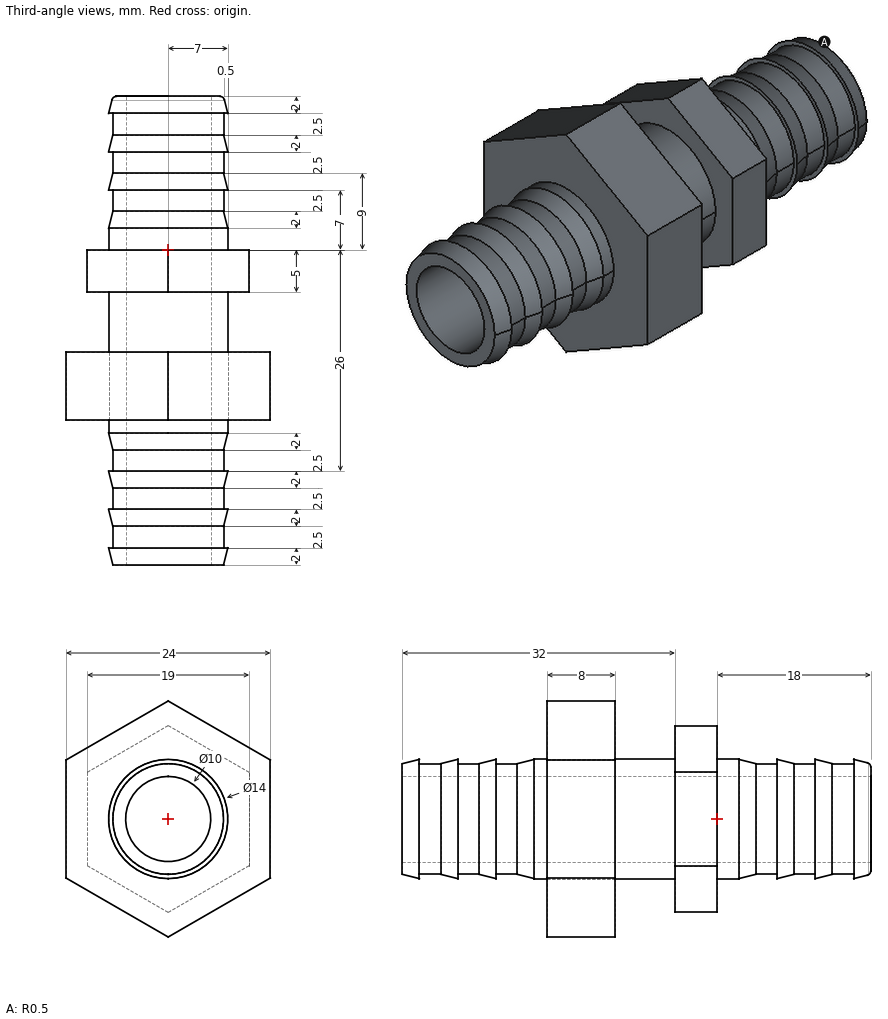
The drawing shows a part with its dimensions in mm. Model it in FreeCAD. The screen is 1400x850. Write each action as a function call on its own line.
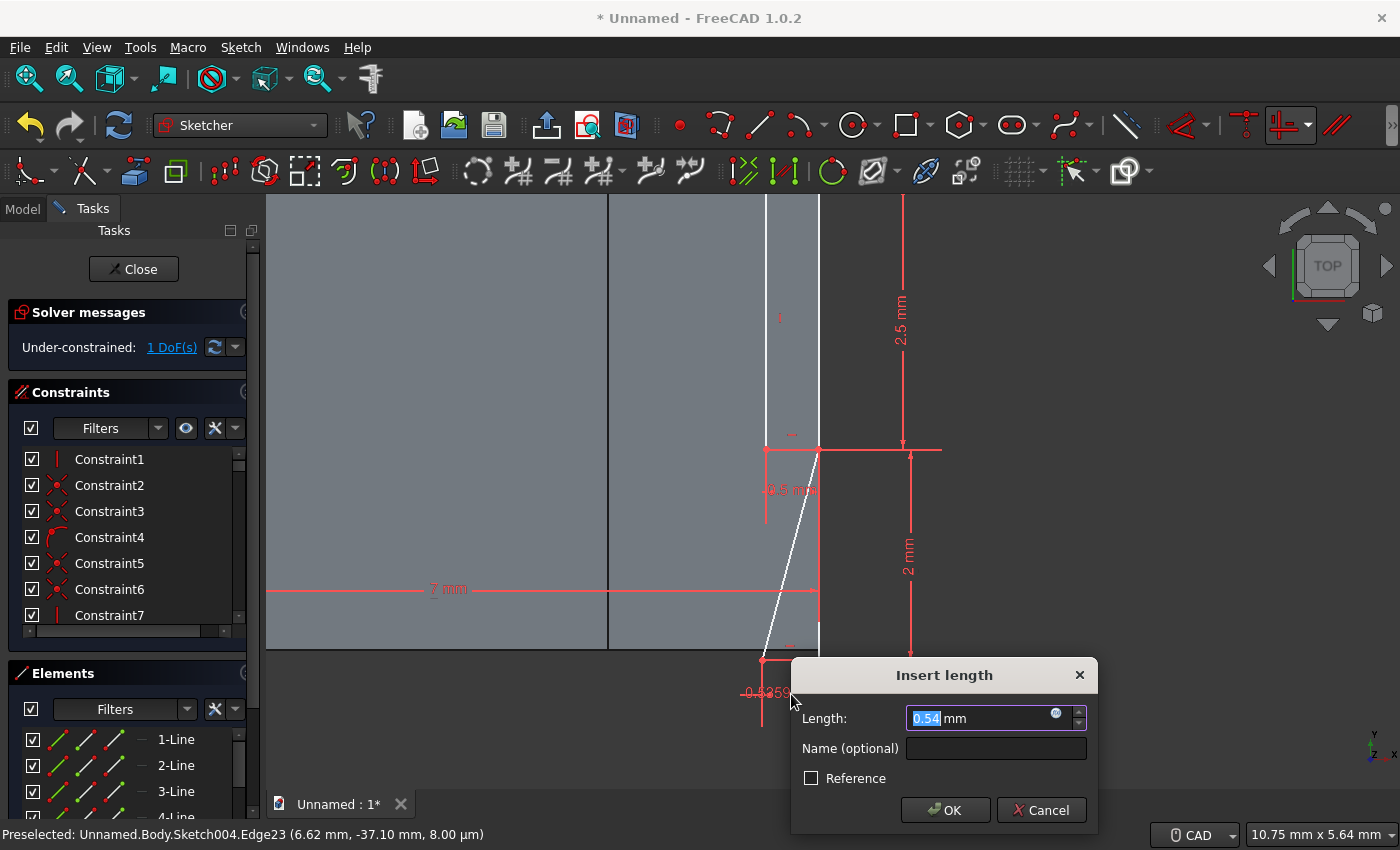
text(0.5)
key(Return)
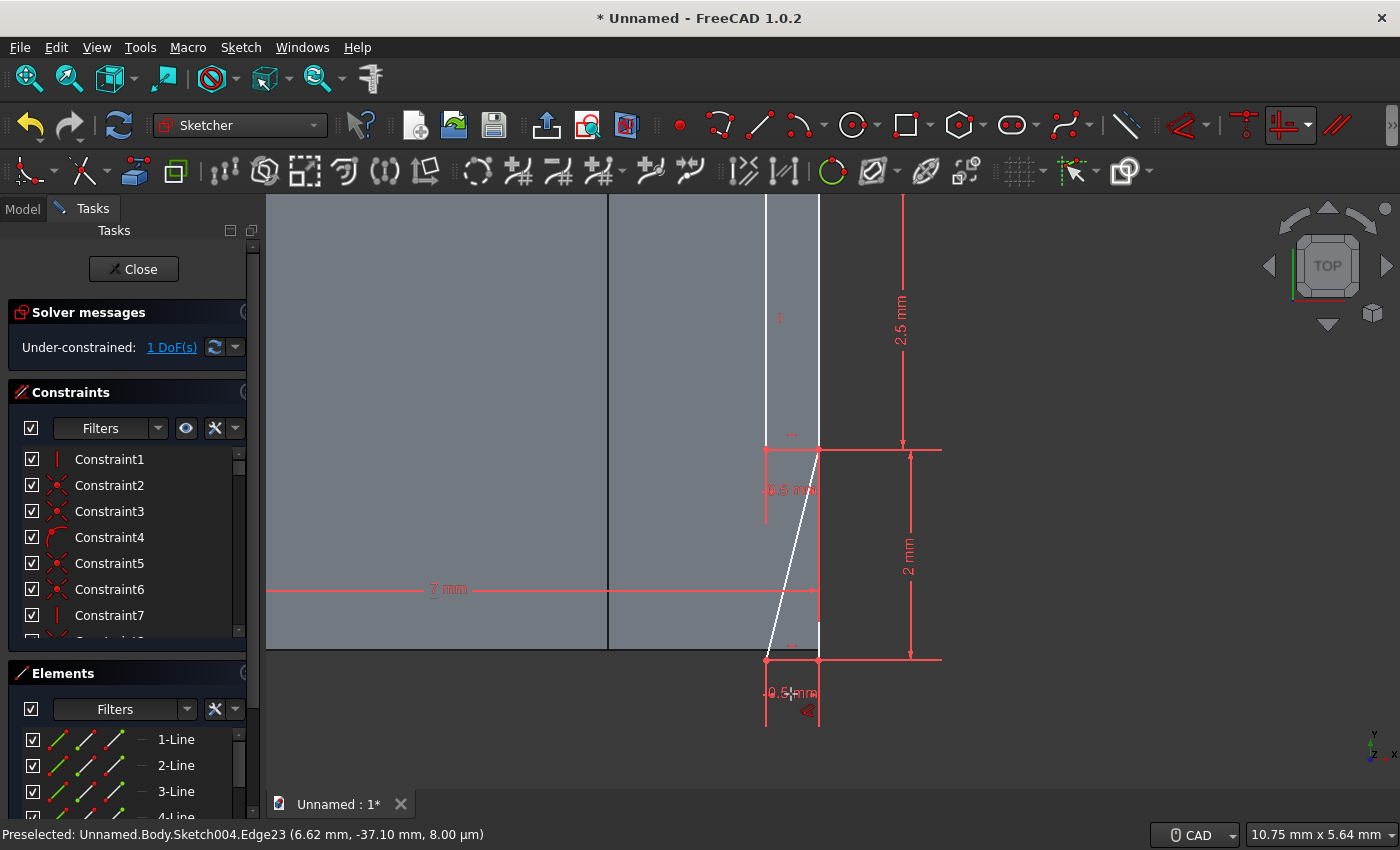
scroll(785, 669, down, 14)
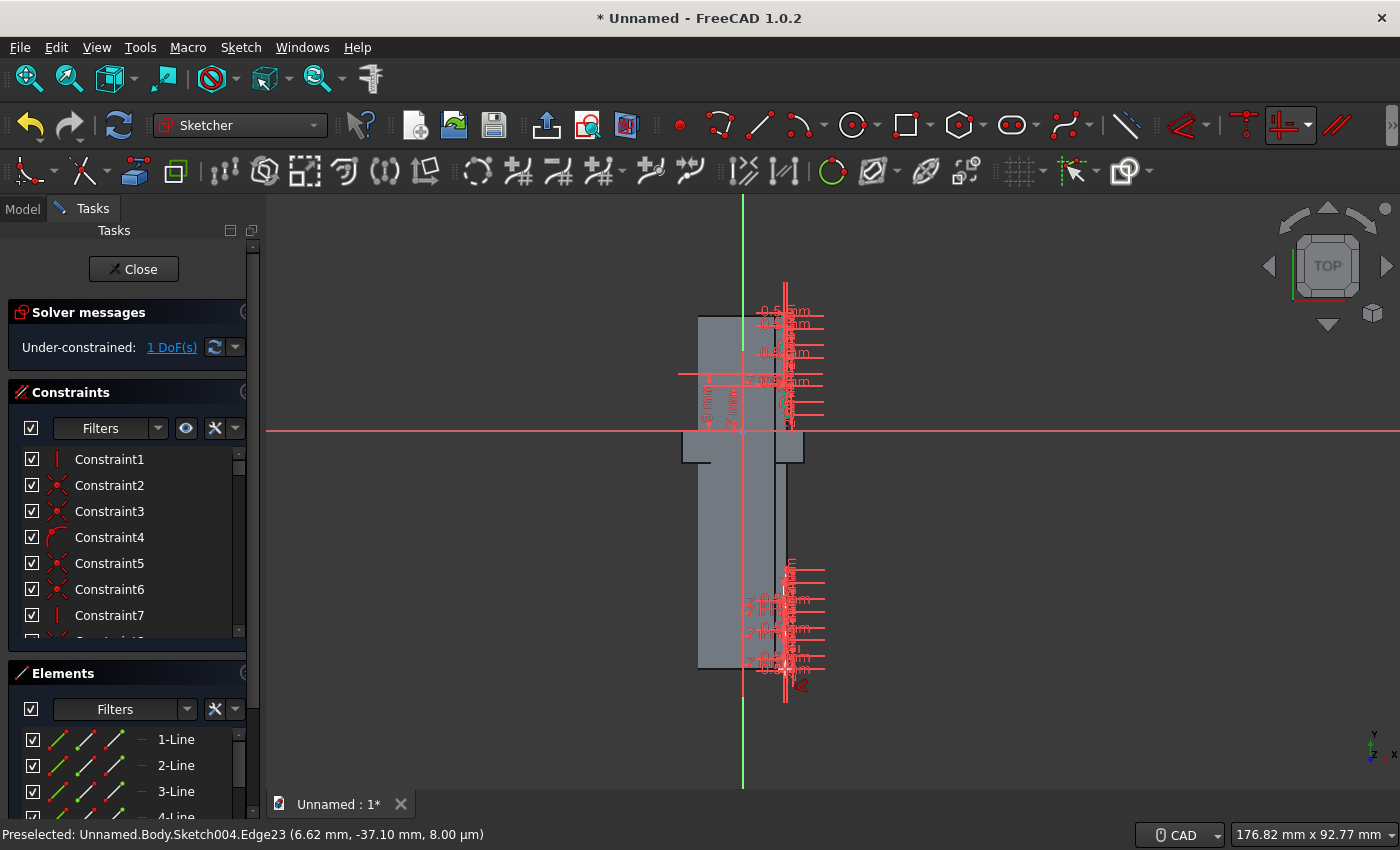
scroll(784, 599, up, 7)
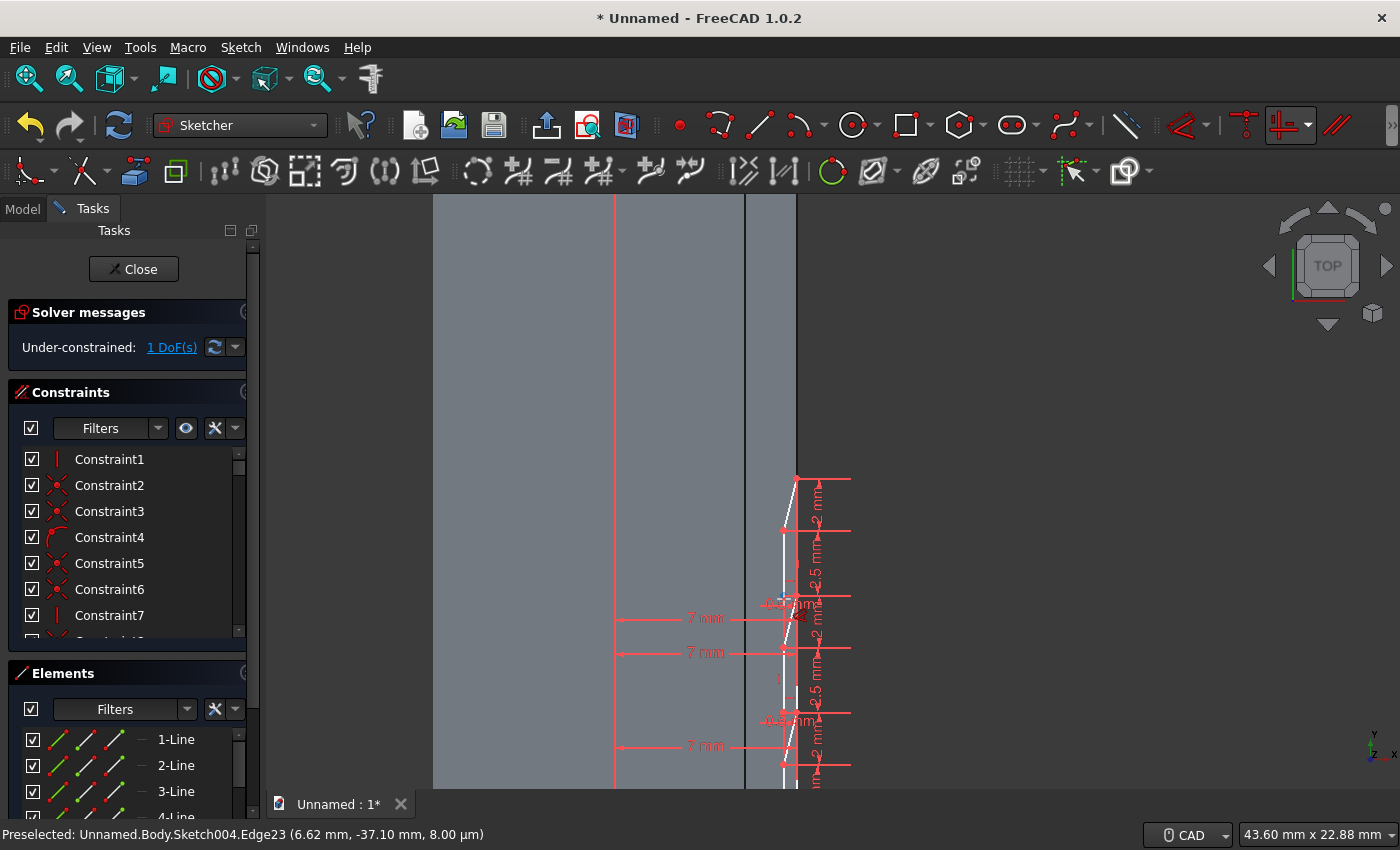
click(784, 596)
click(581, 409)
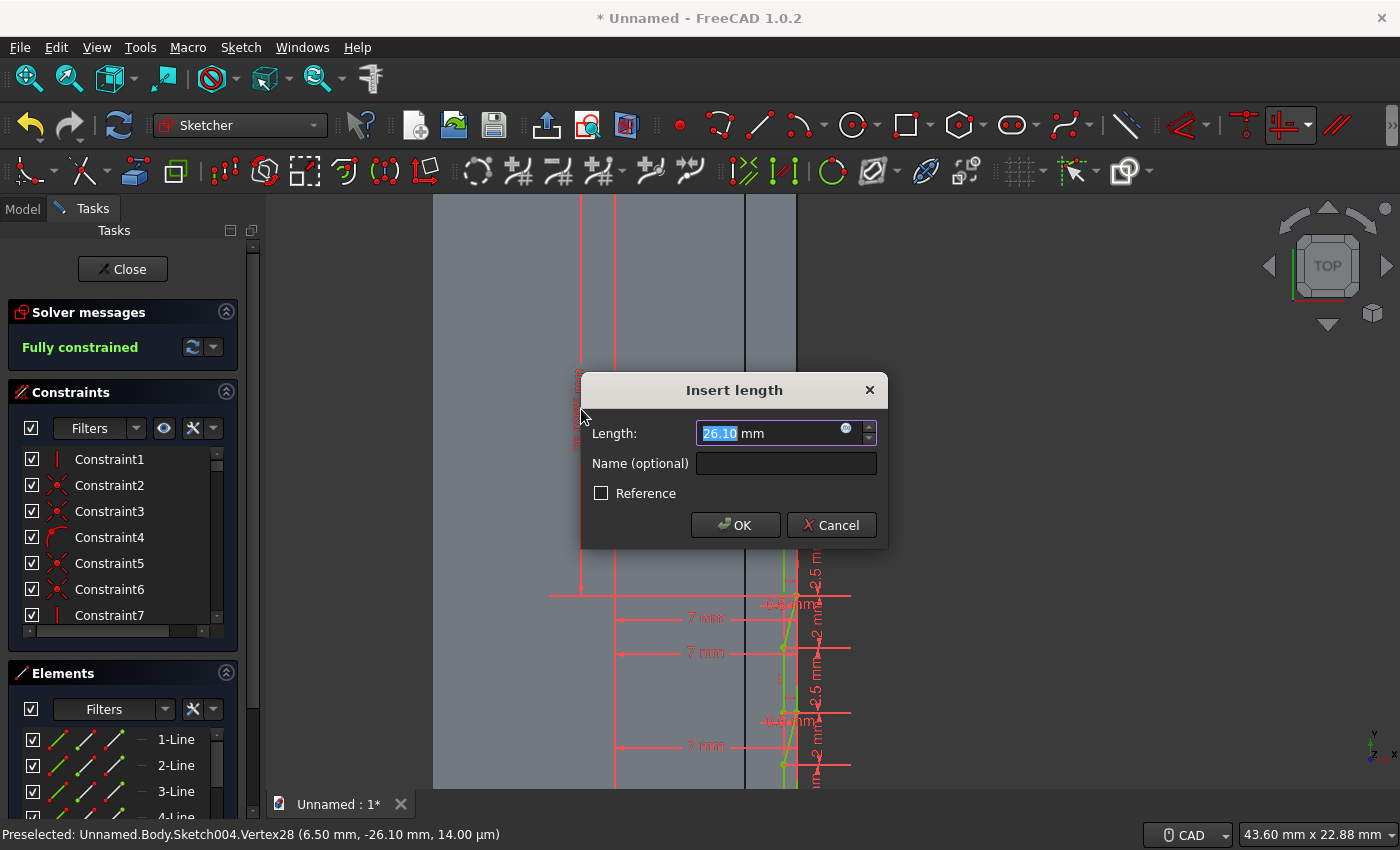
text(26)
key(Return)
key(Escape)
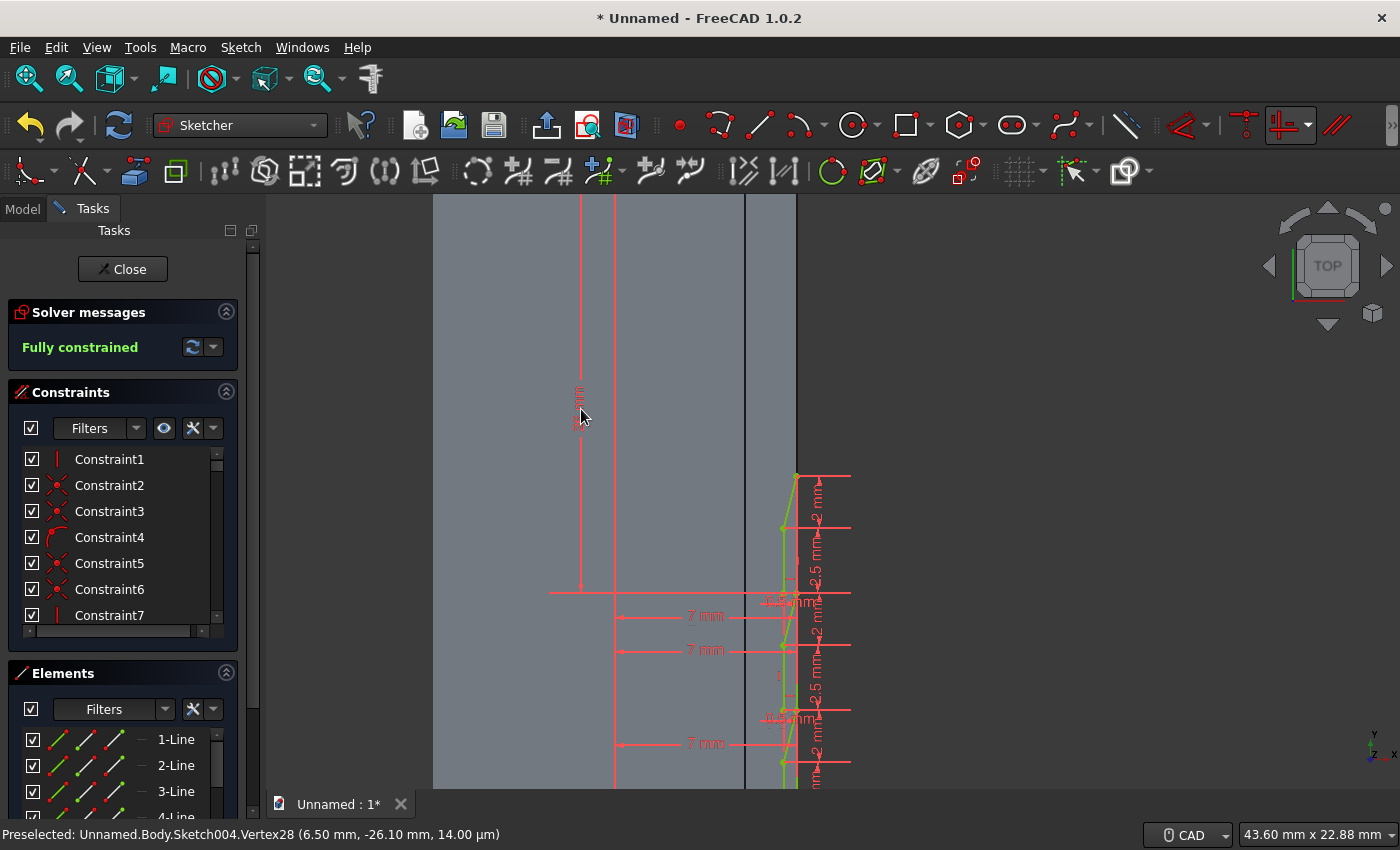
click(123, 269)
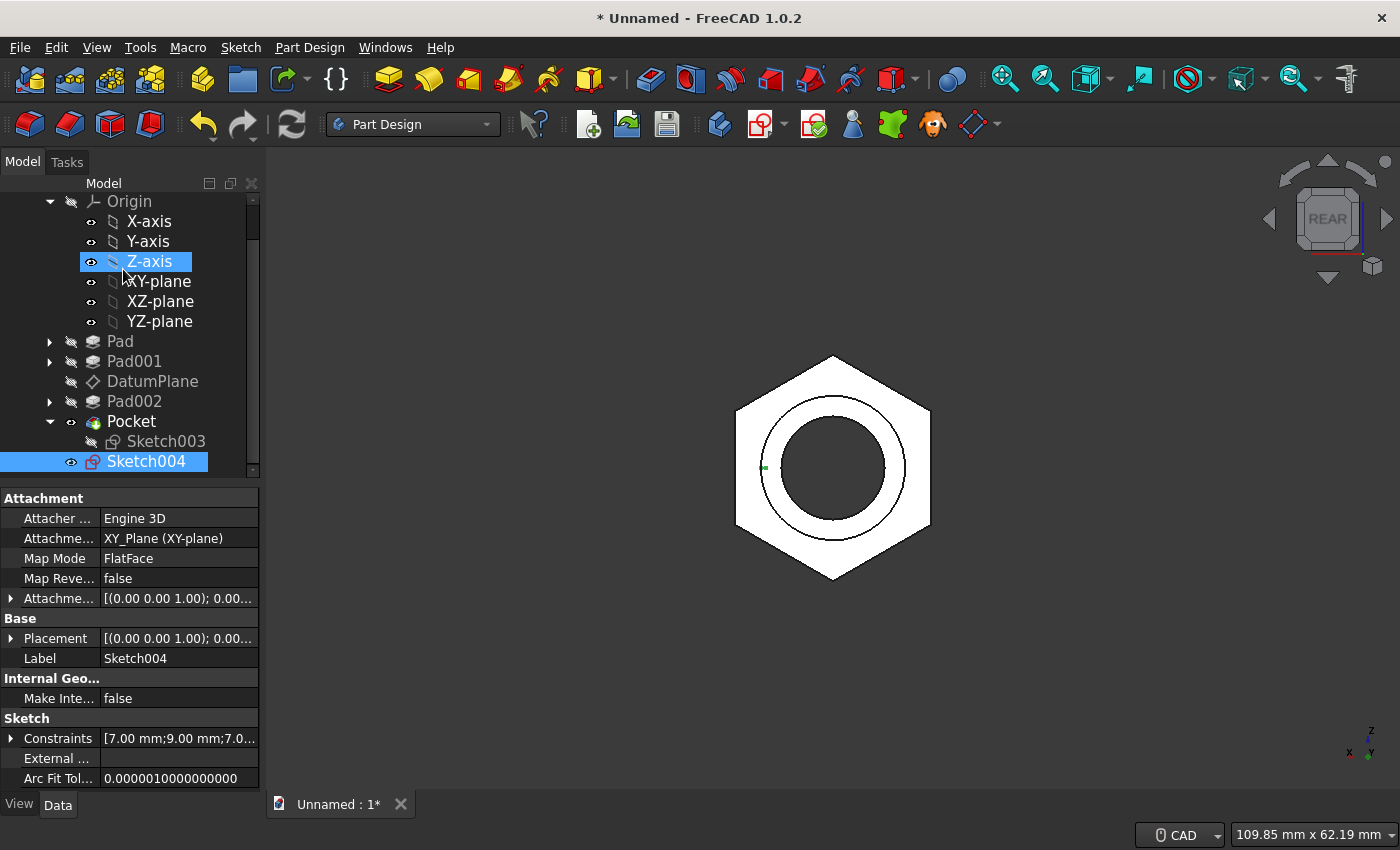
click(732, 80)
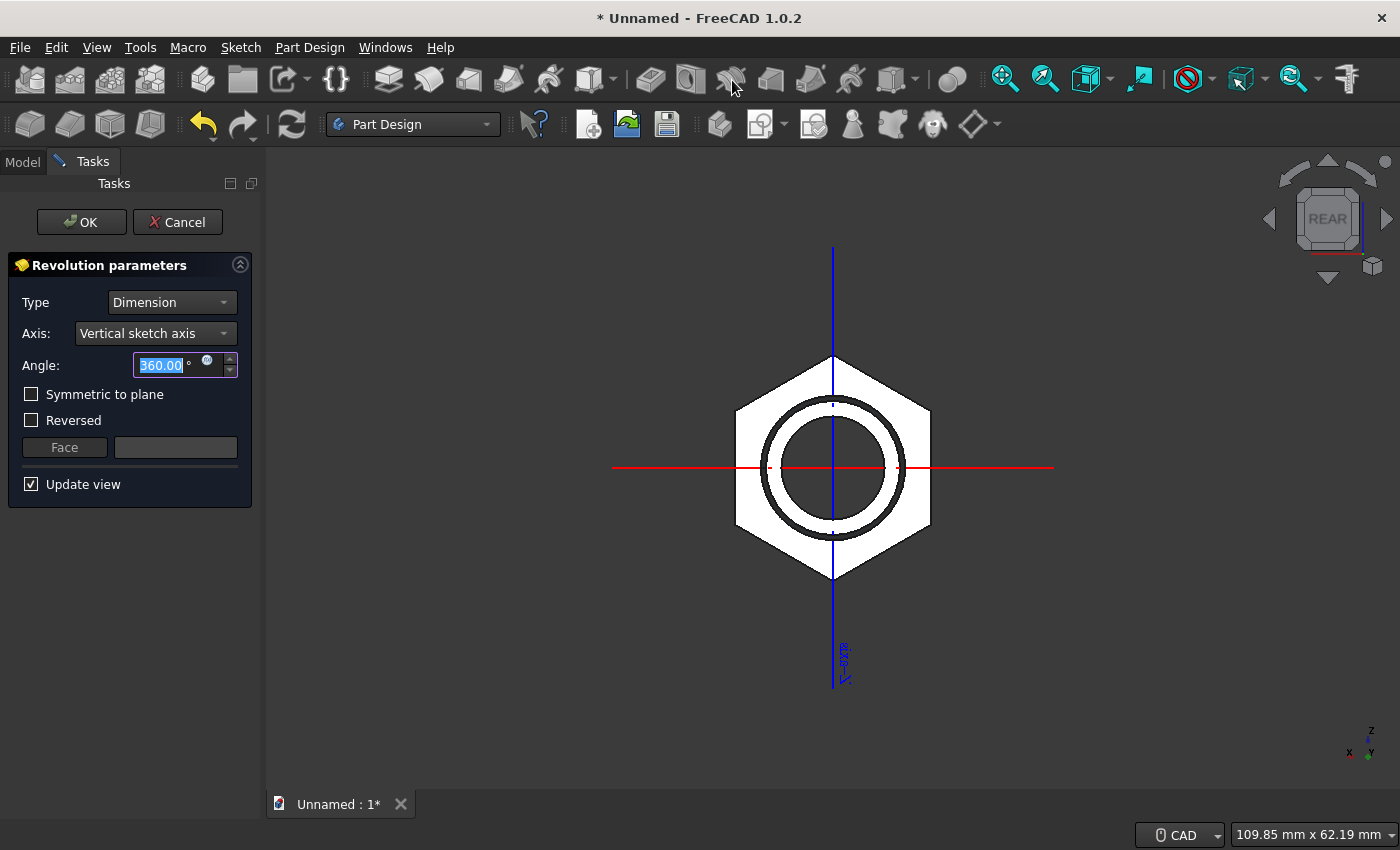
click(82, 222)